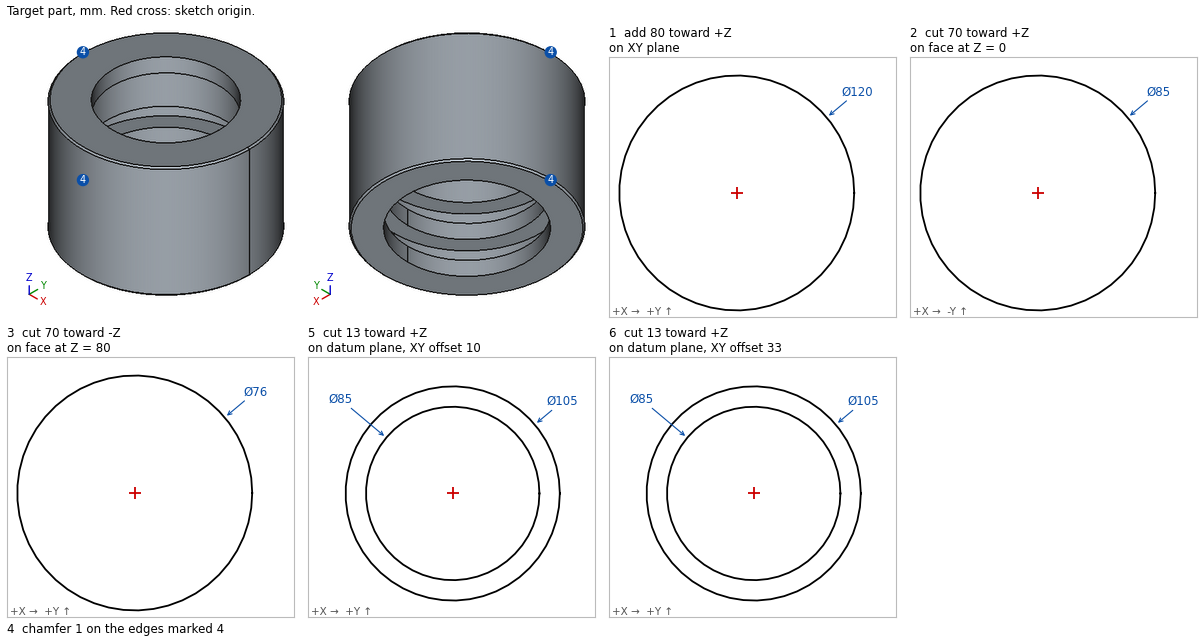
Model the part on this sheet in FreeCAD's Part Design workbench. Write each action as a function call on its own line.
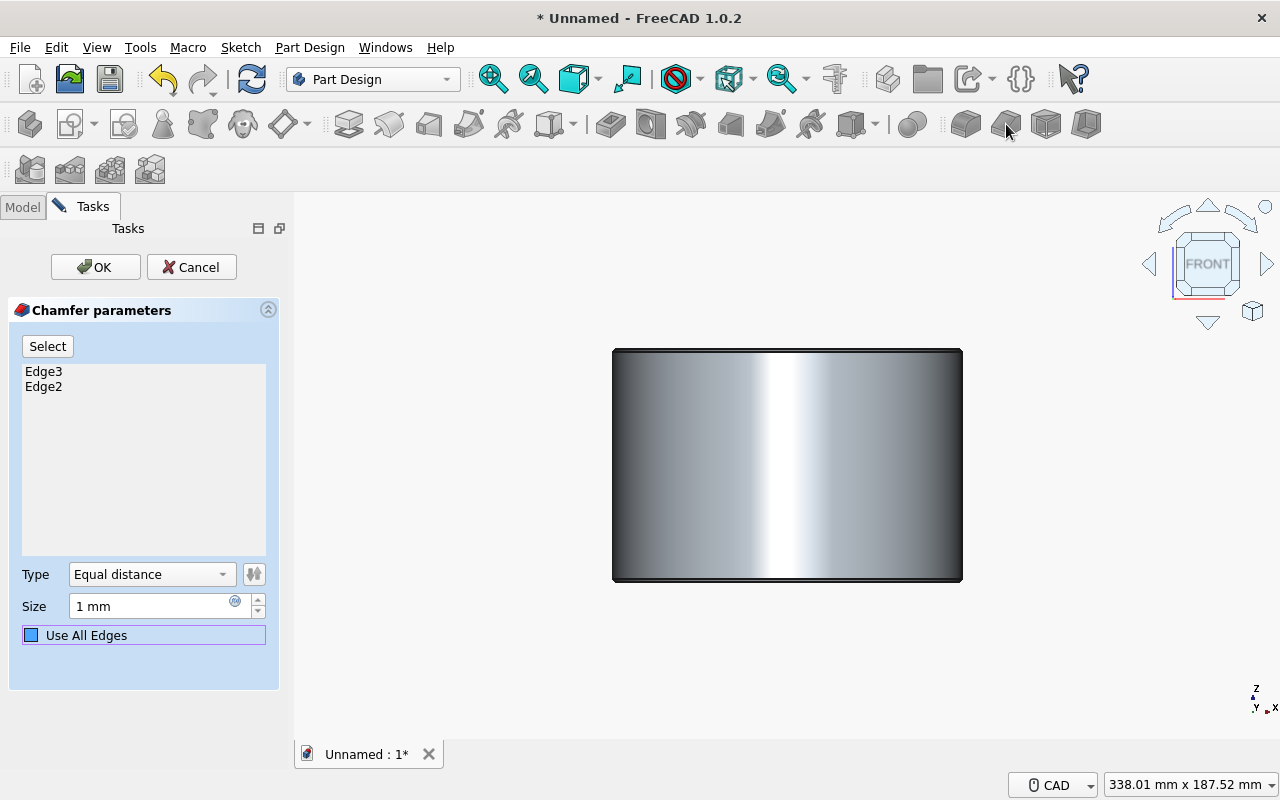
click(96, 267)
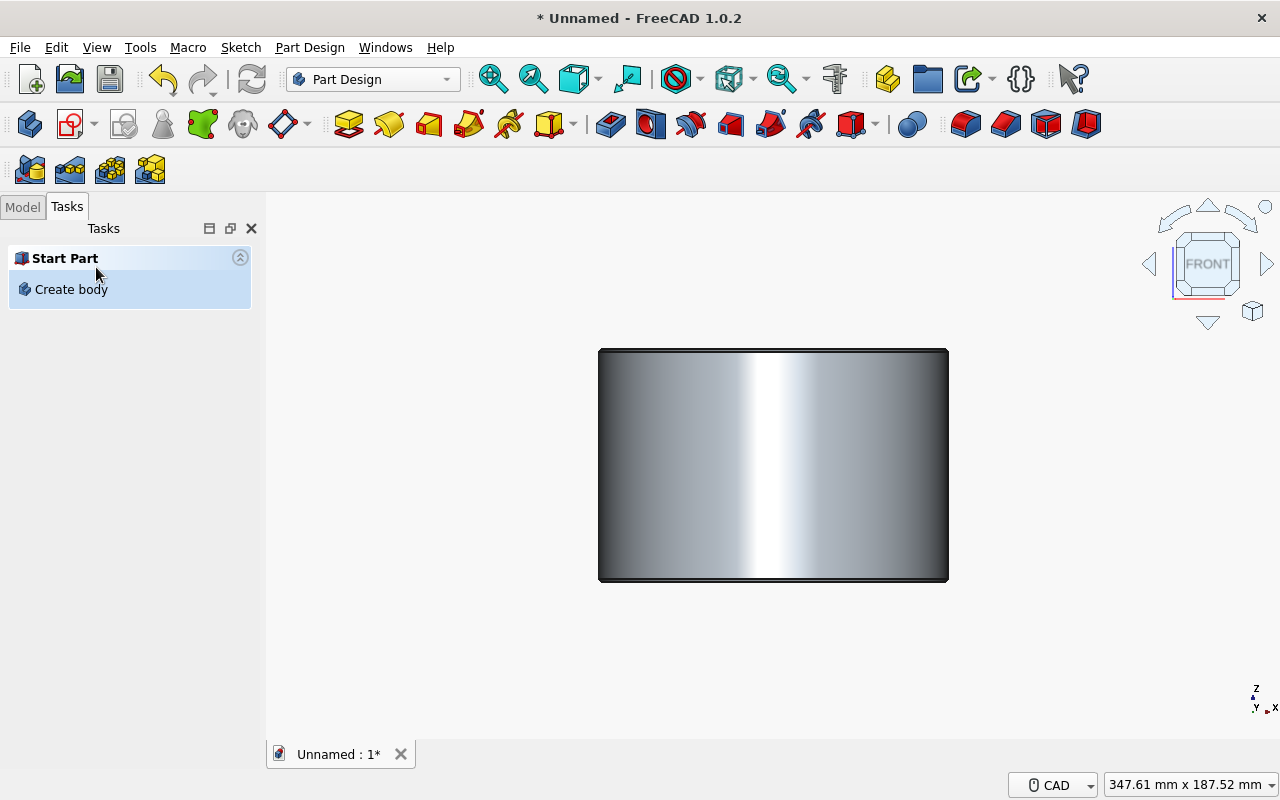
click(494, 80)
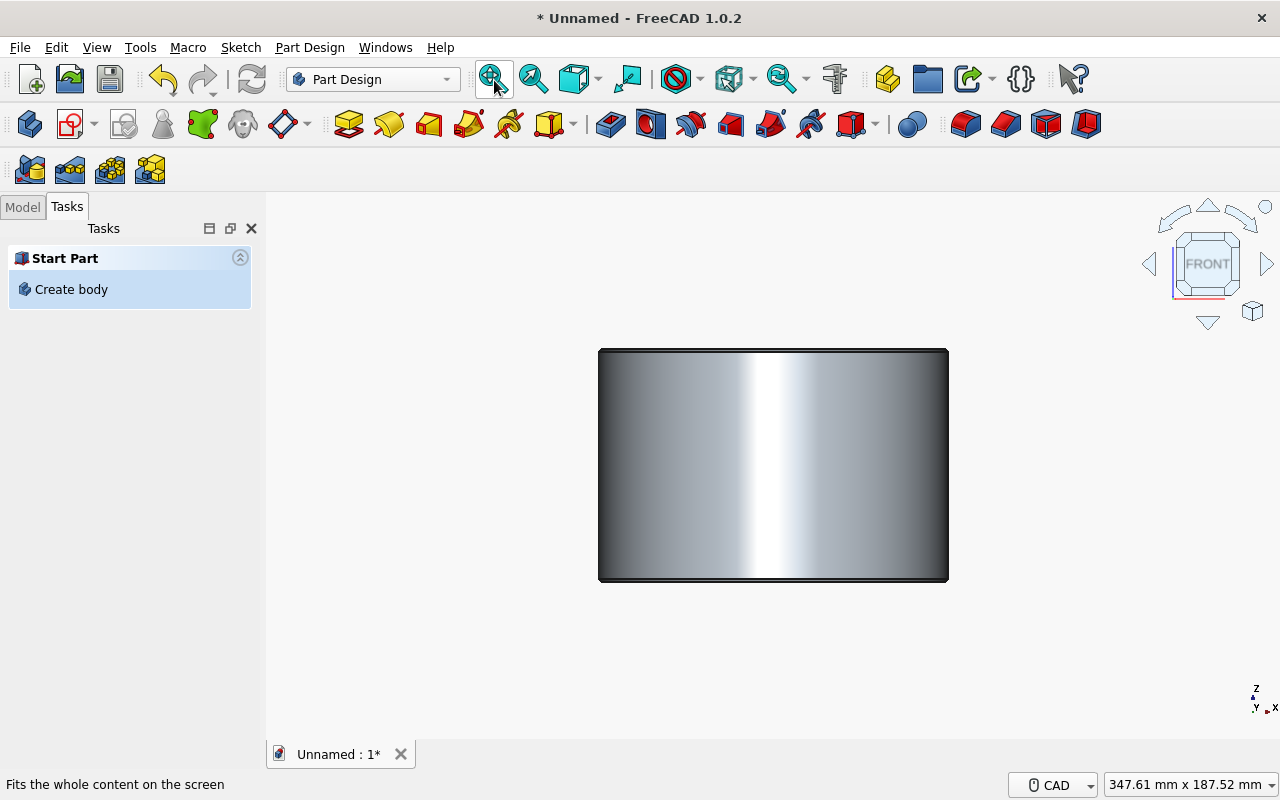
click(23, 206)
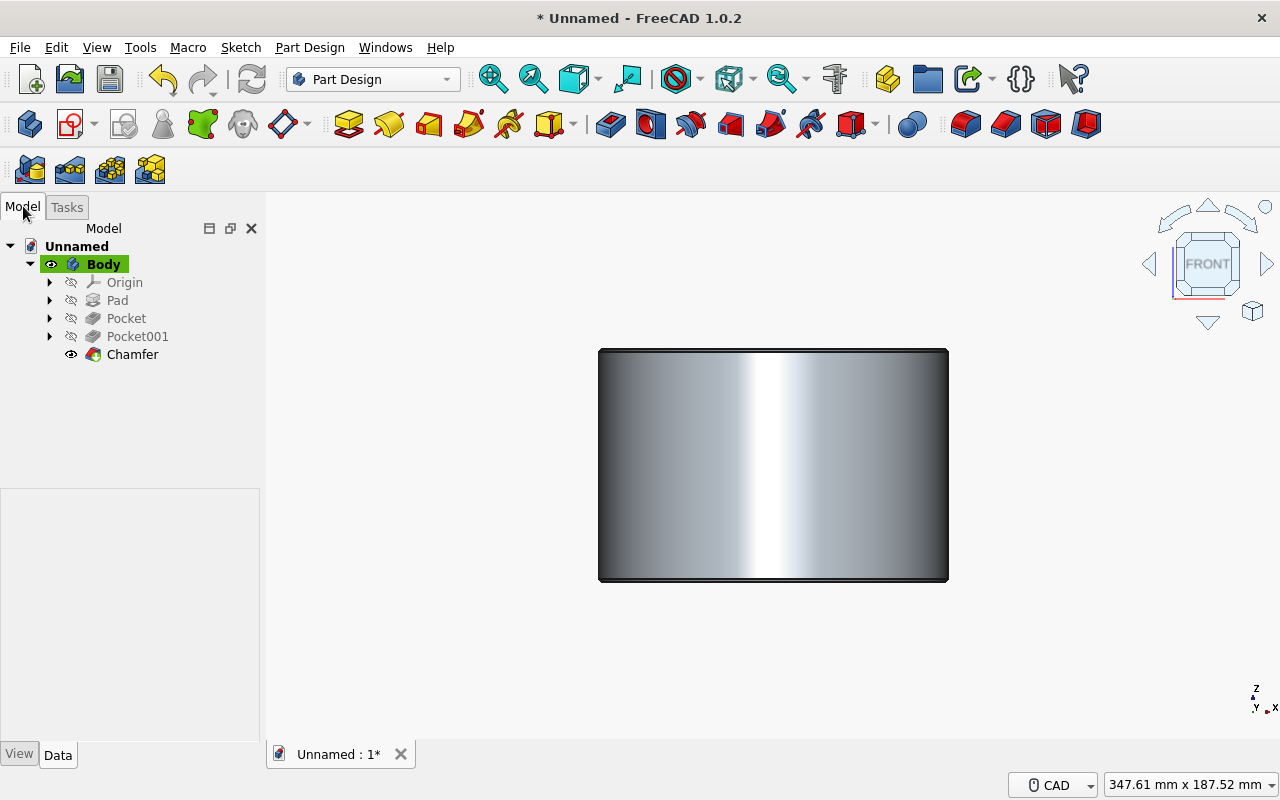
click(50, 282)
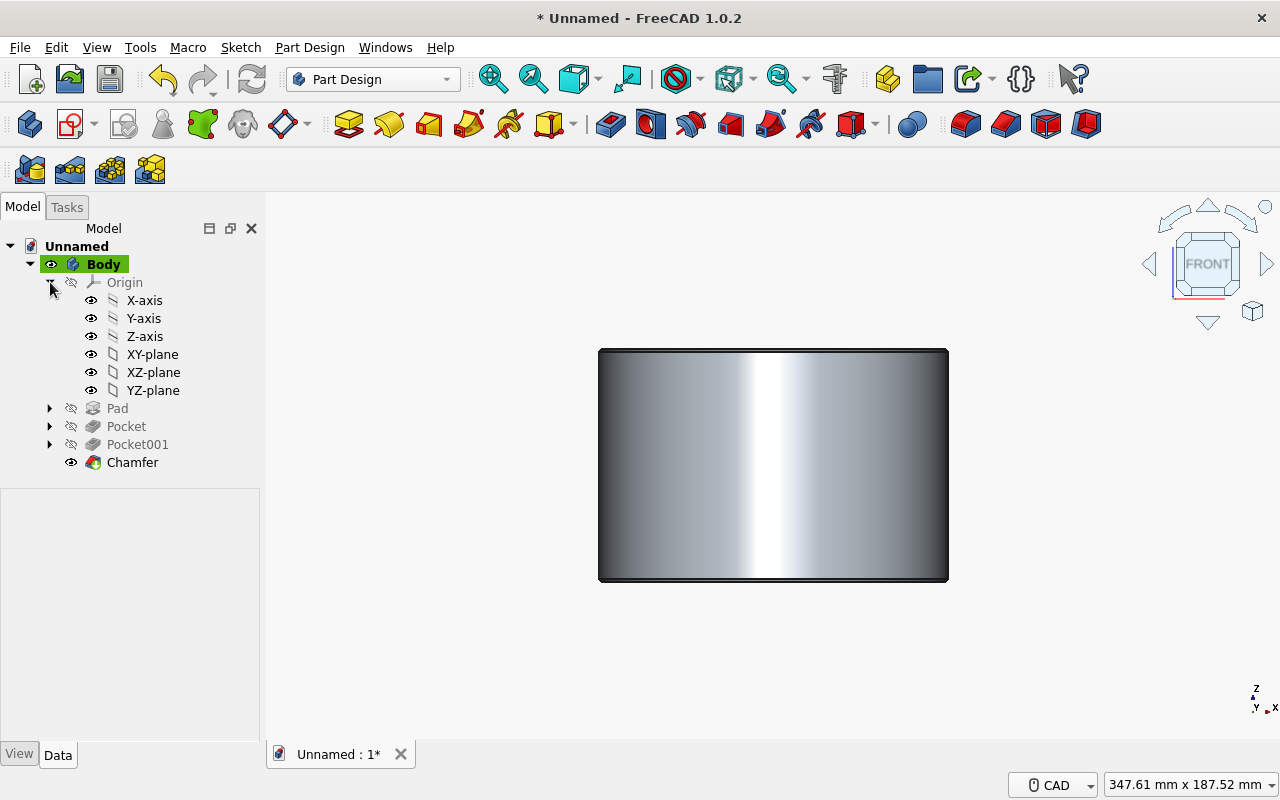
click(136, 354)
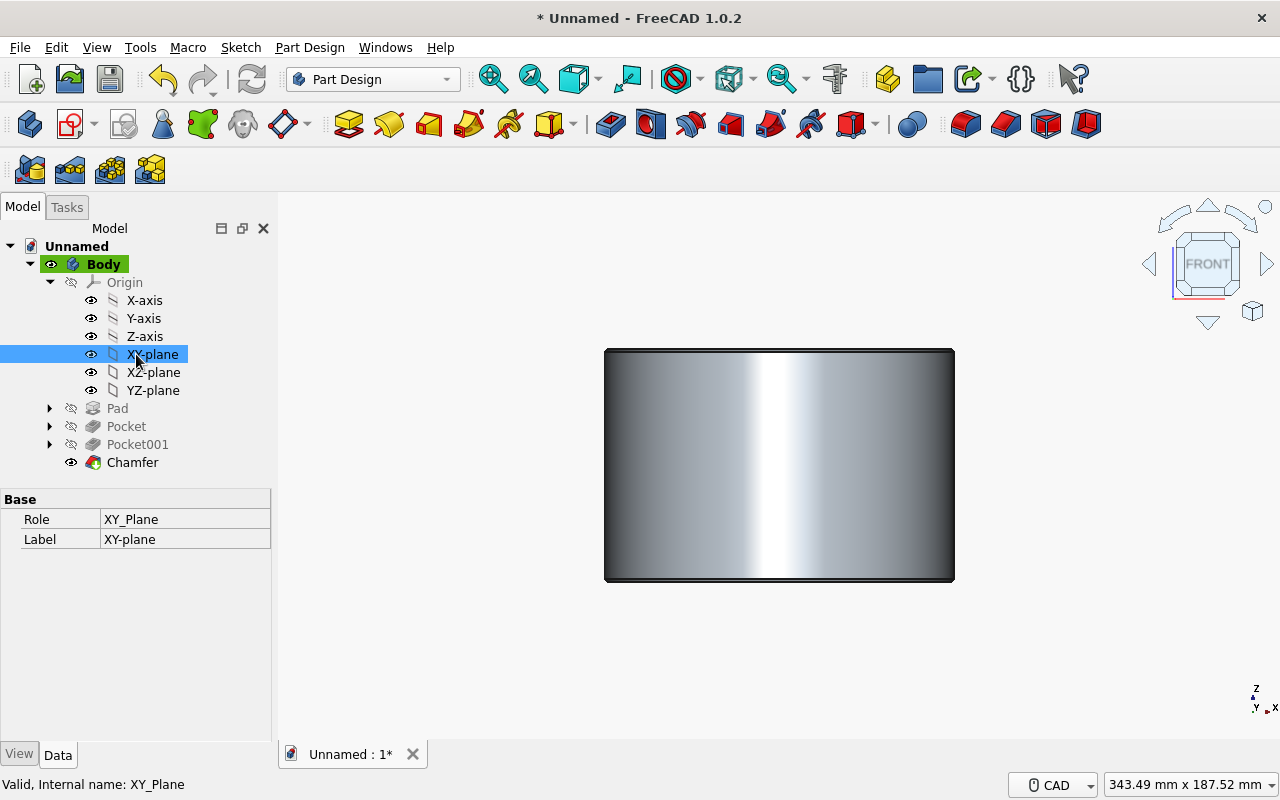
click(284, 124)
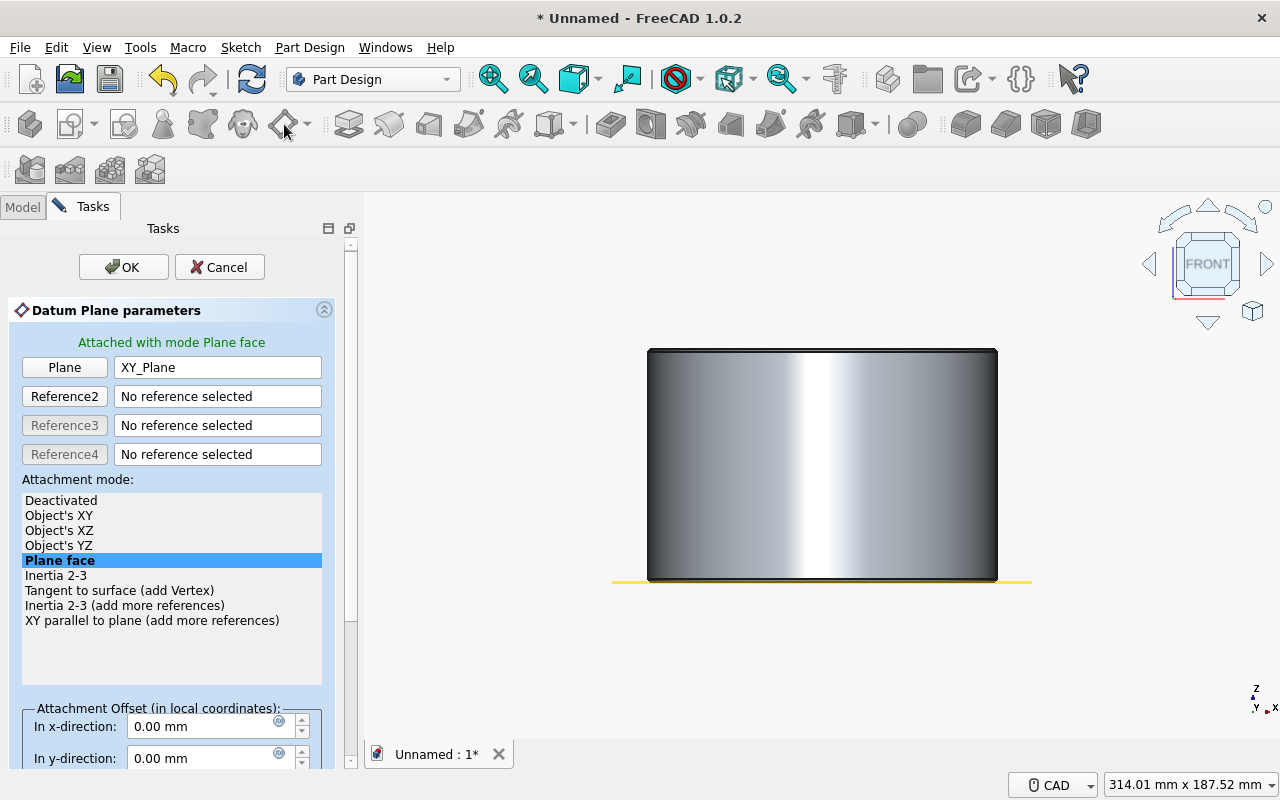
scroll(351, 503, down, 2)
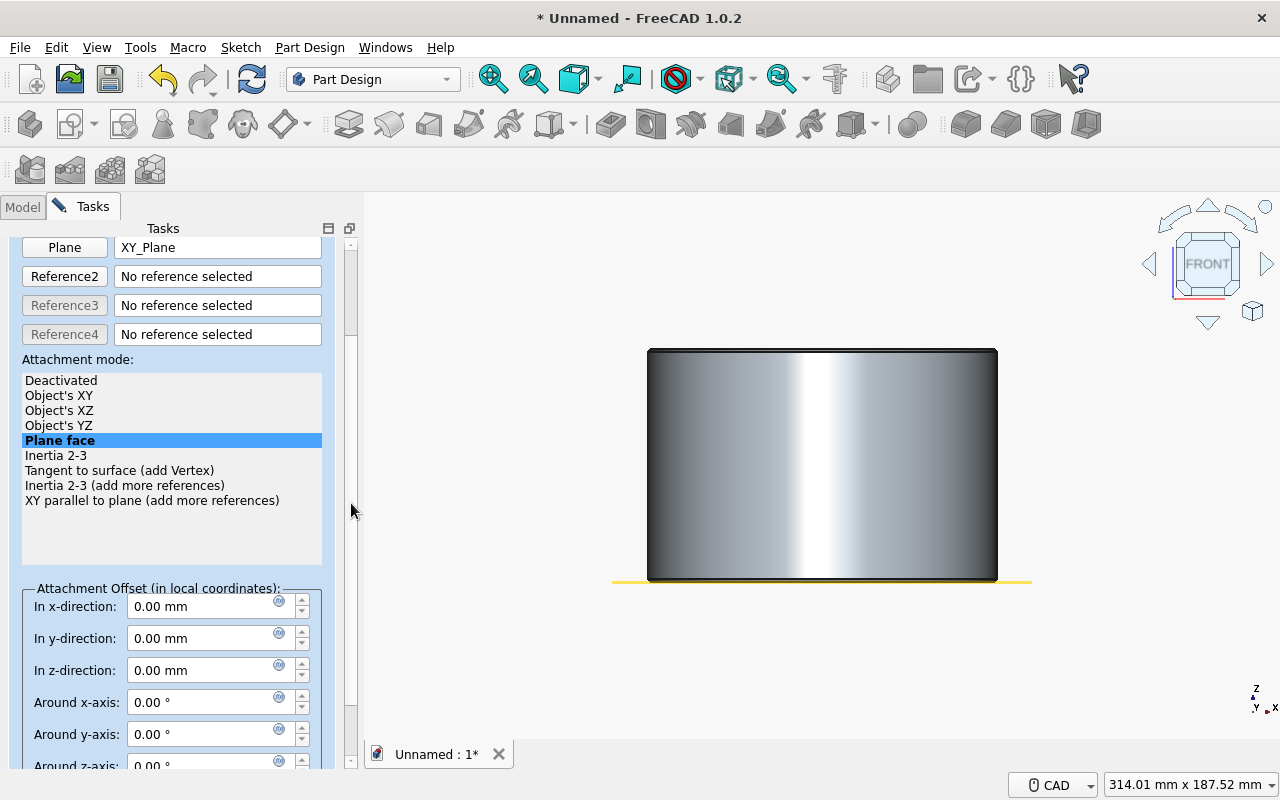
triple_click(210, 670)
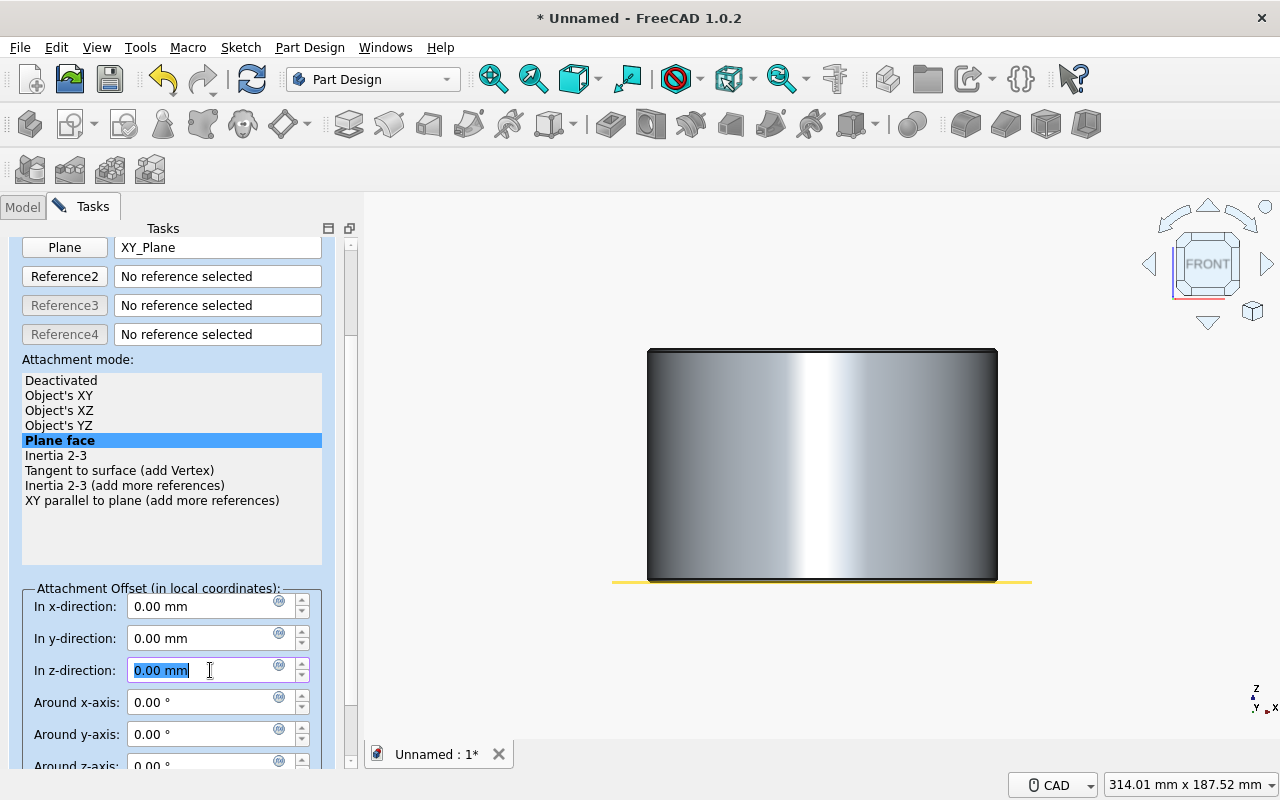
text(10)
key(Tab)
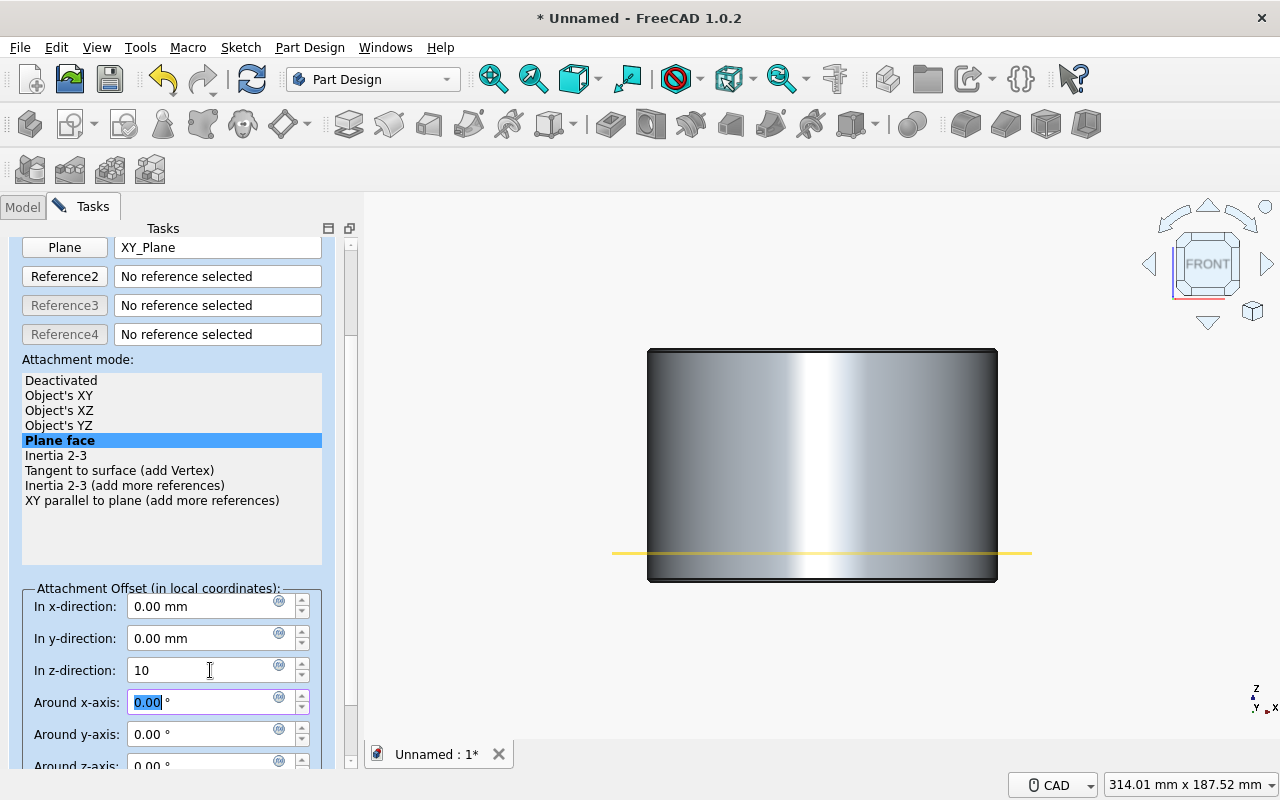
scroll(351, 503, up, 3)